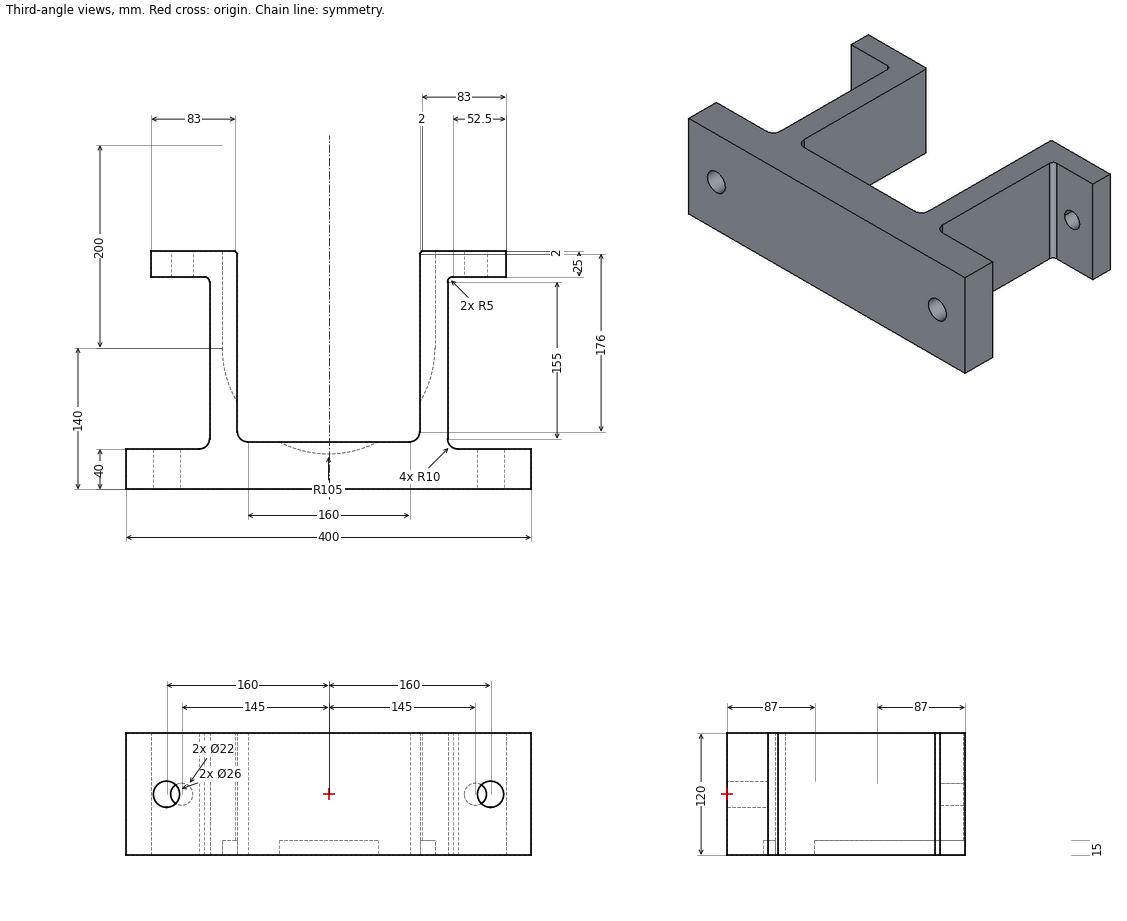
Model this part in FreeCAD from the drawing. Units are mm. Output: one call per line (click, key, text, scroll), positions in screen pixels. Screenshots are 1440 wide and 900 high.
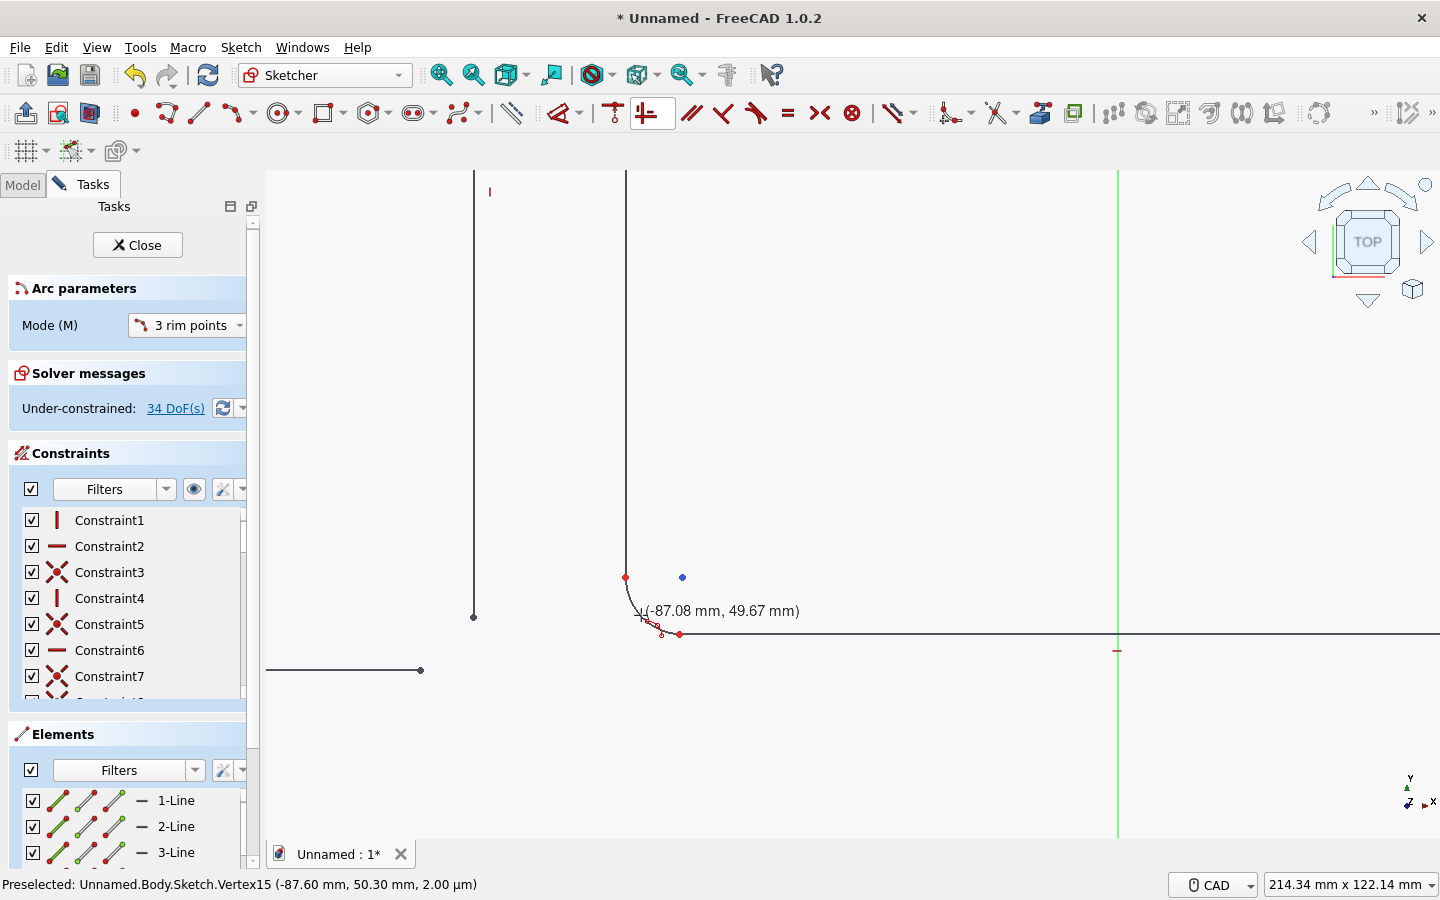
scroll(641, 617, down, 6)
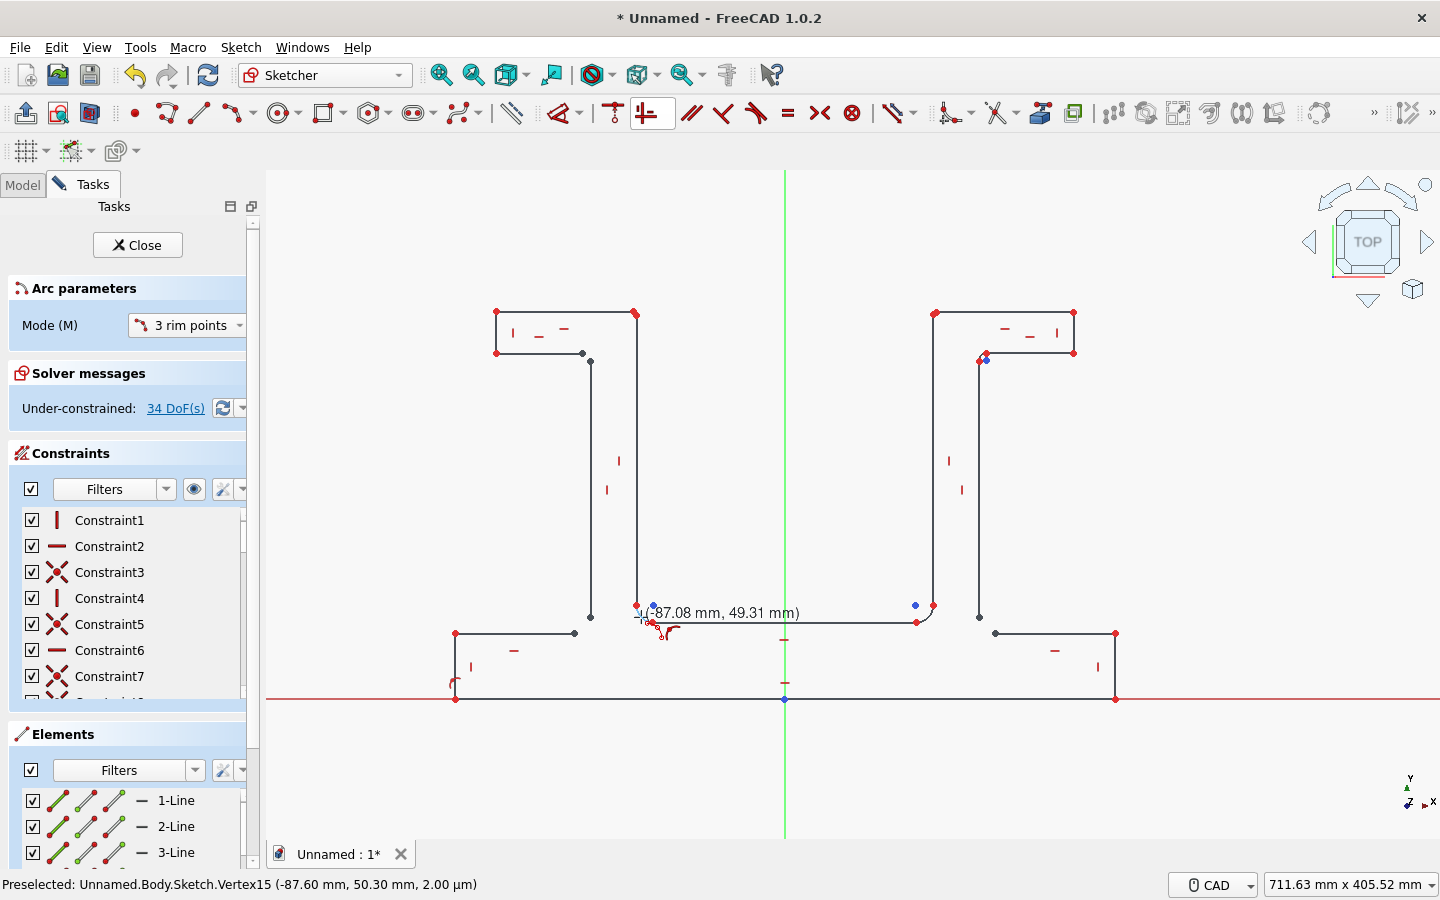
scroll(583, 353, up, 2)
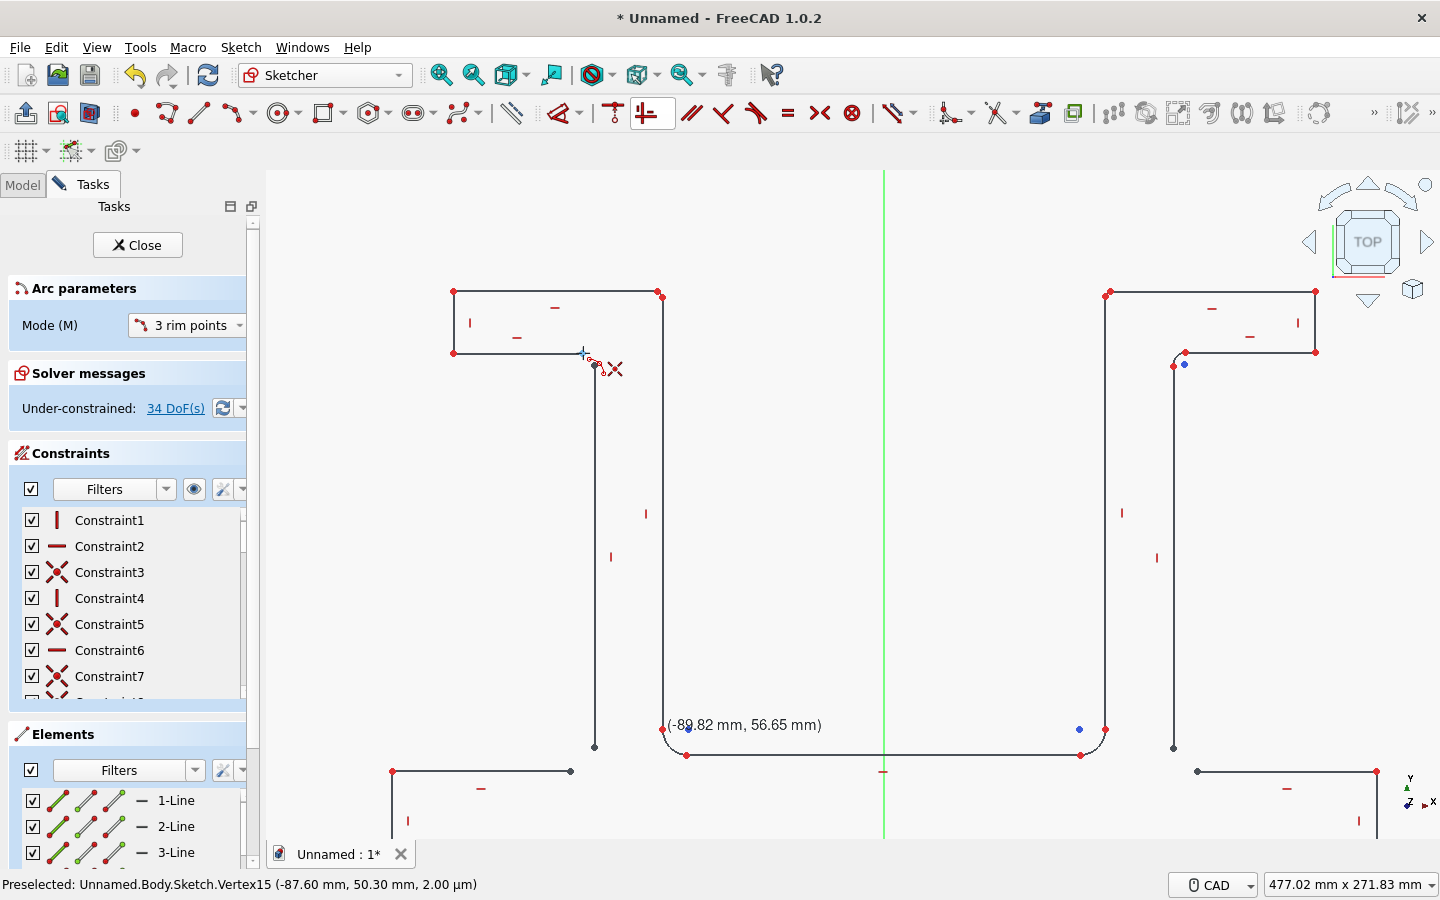
click(582, 354)
click(595, 365)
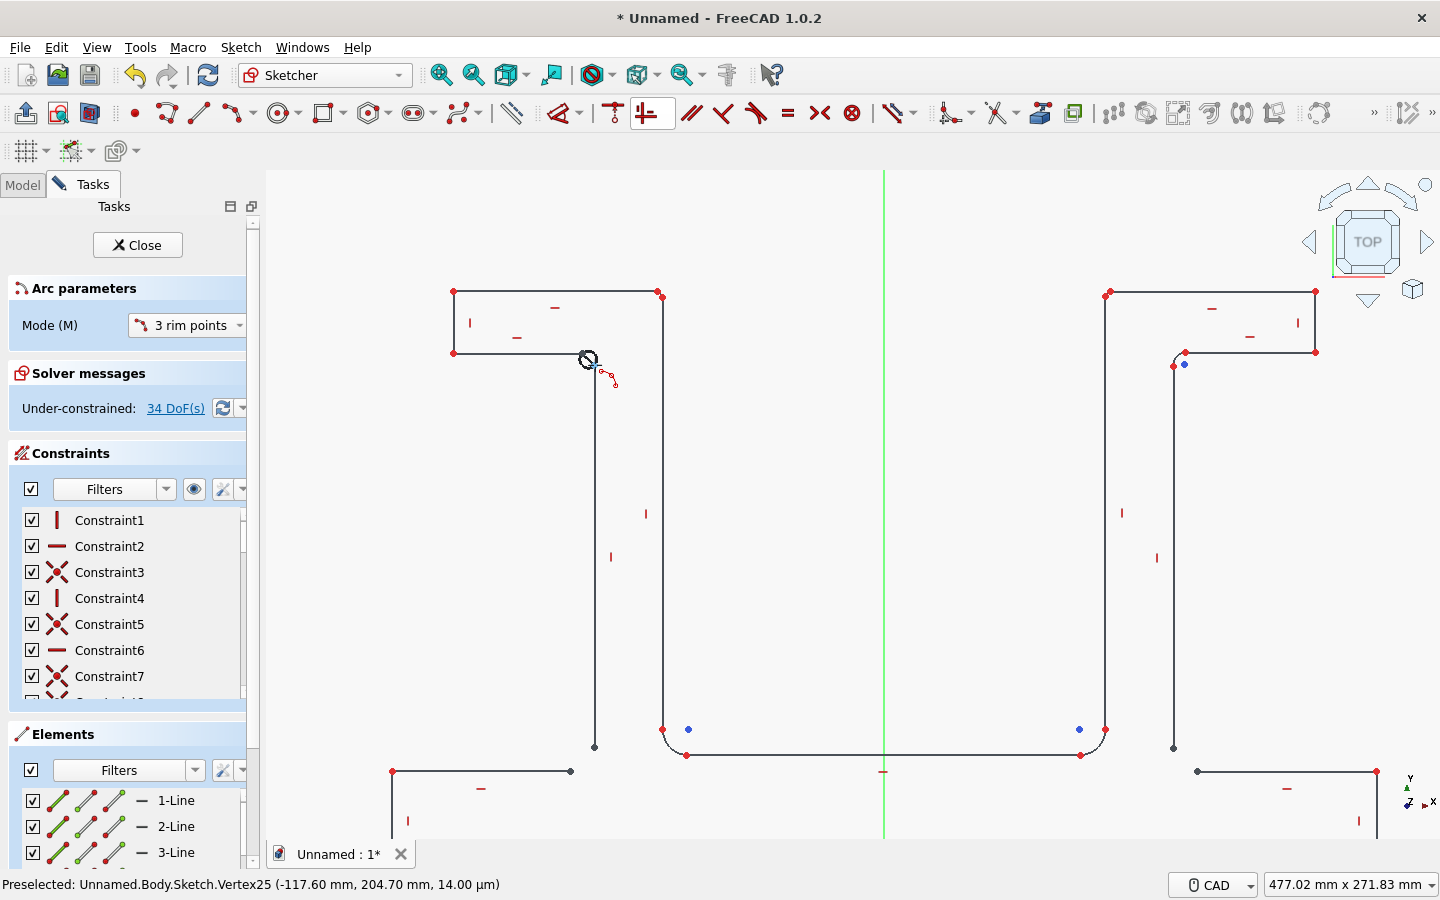
scroll(591, 356, up, 8)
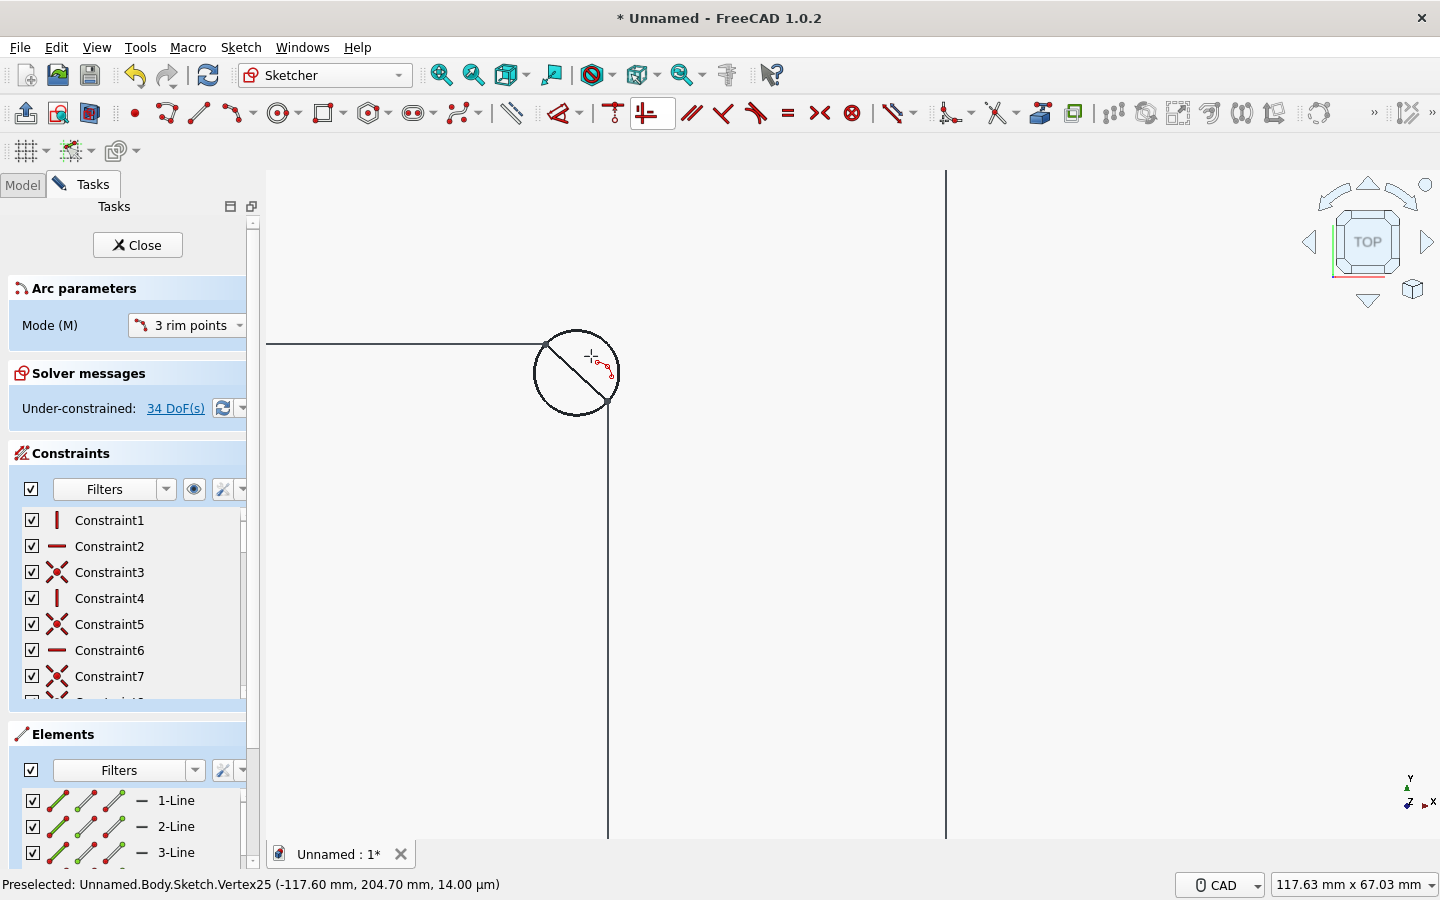
click(591, 355)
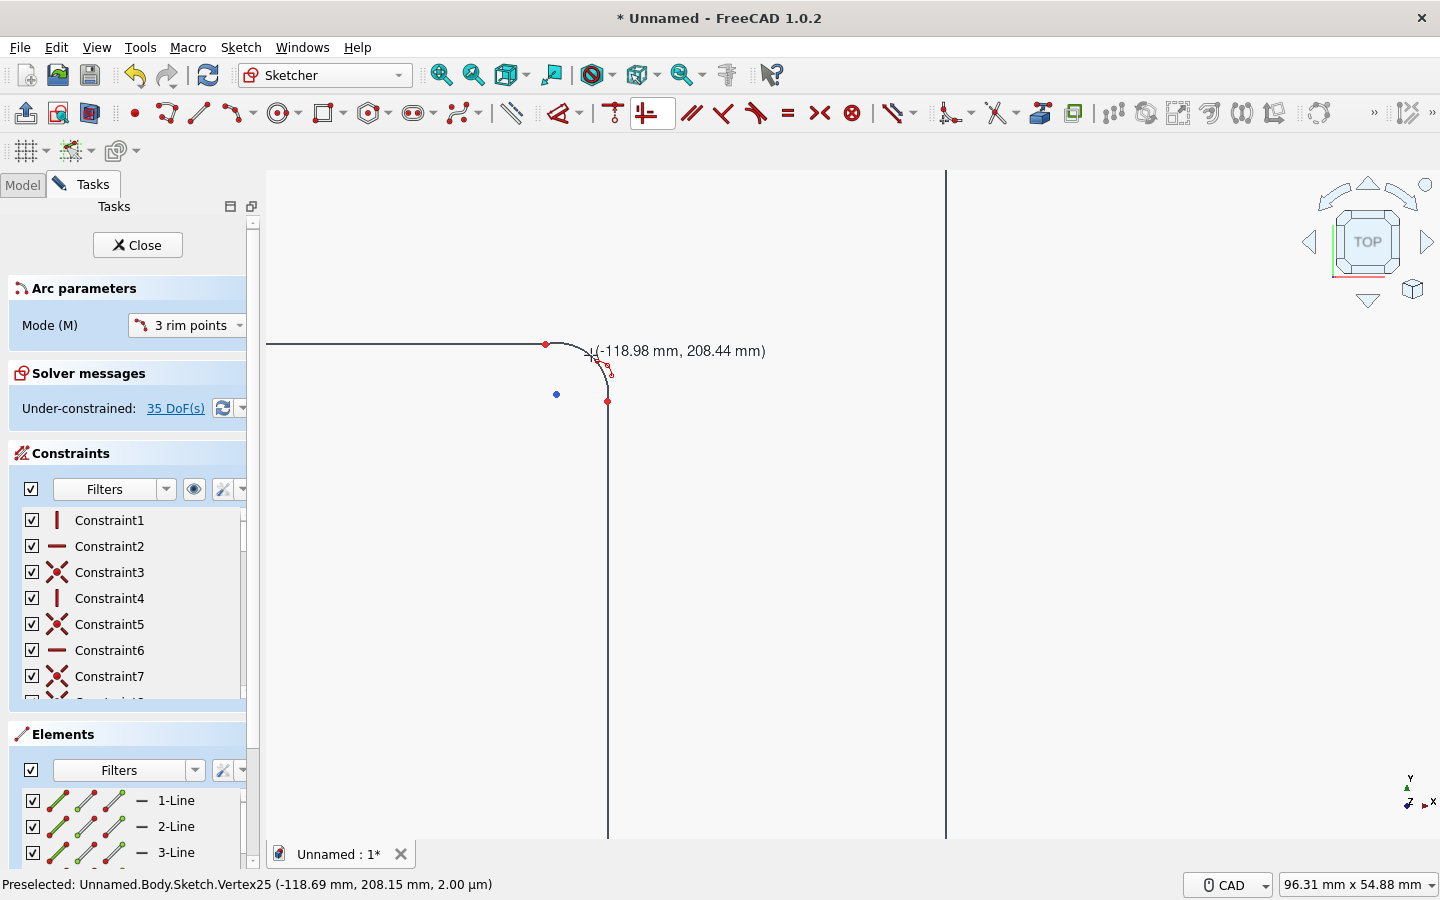
scroll(588, 354, down, 10)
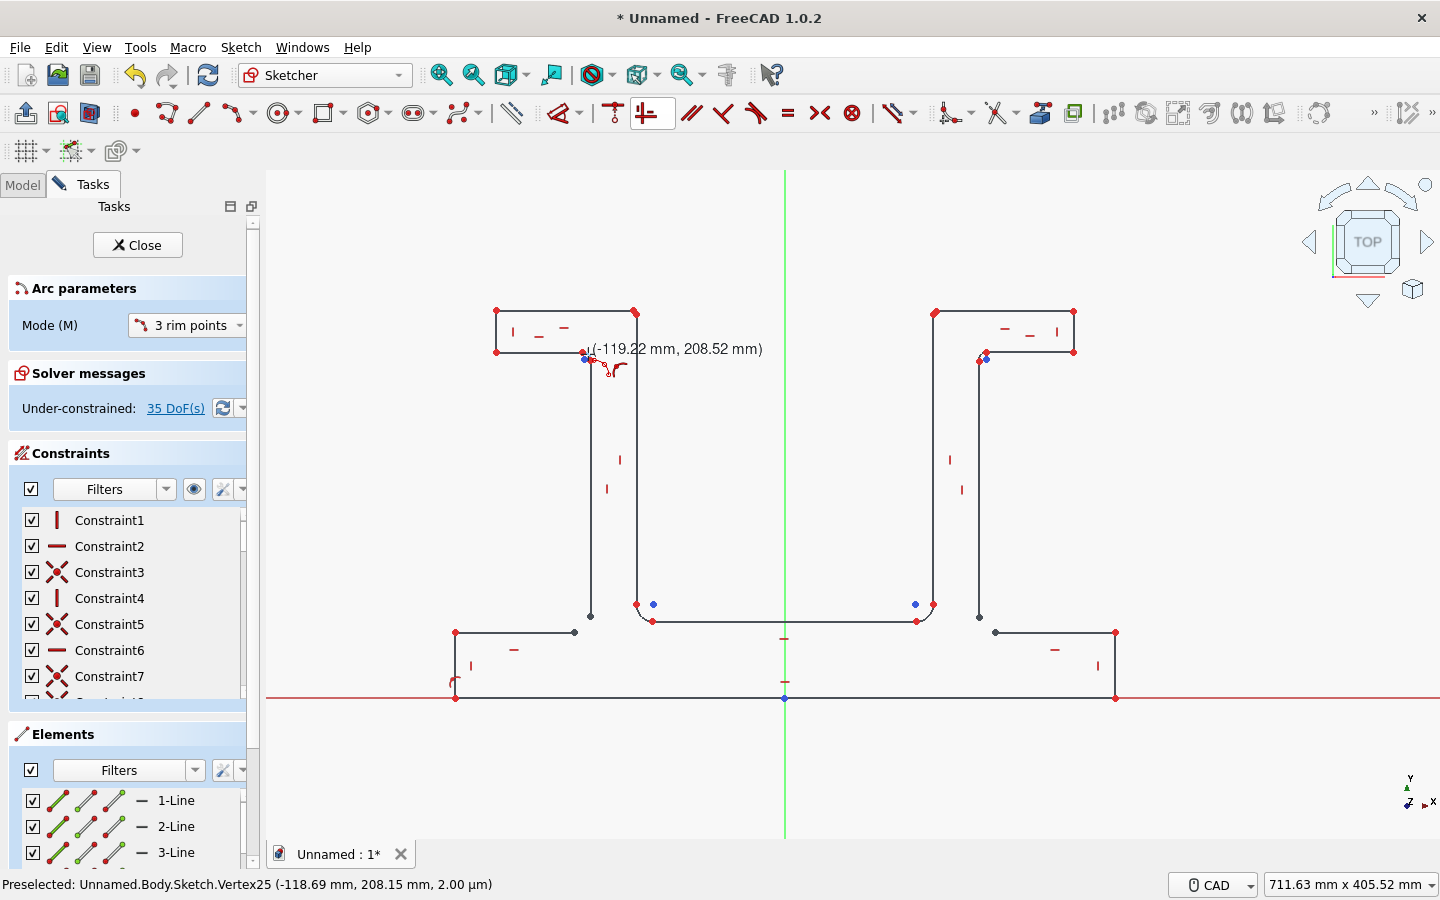
click(591, 617)
click(575, 633)